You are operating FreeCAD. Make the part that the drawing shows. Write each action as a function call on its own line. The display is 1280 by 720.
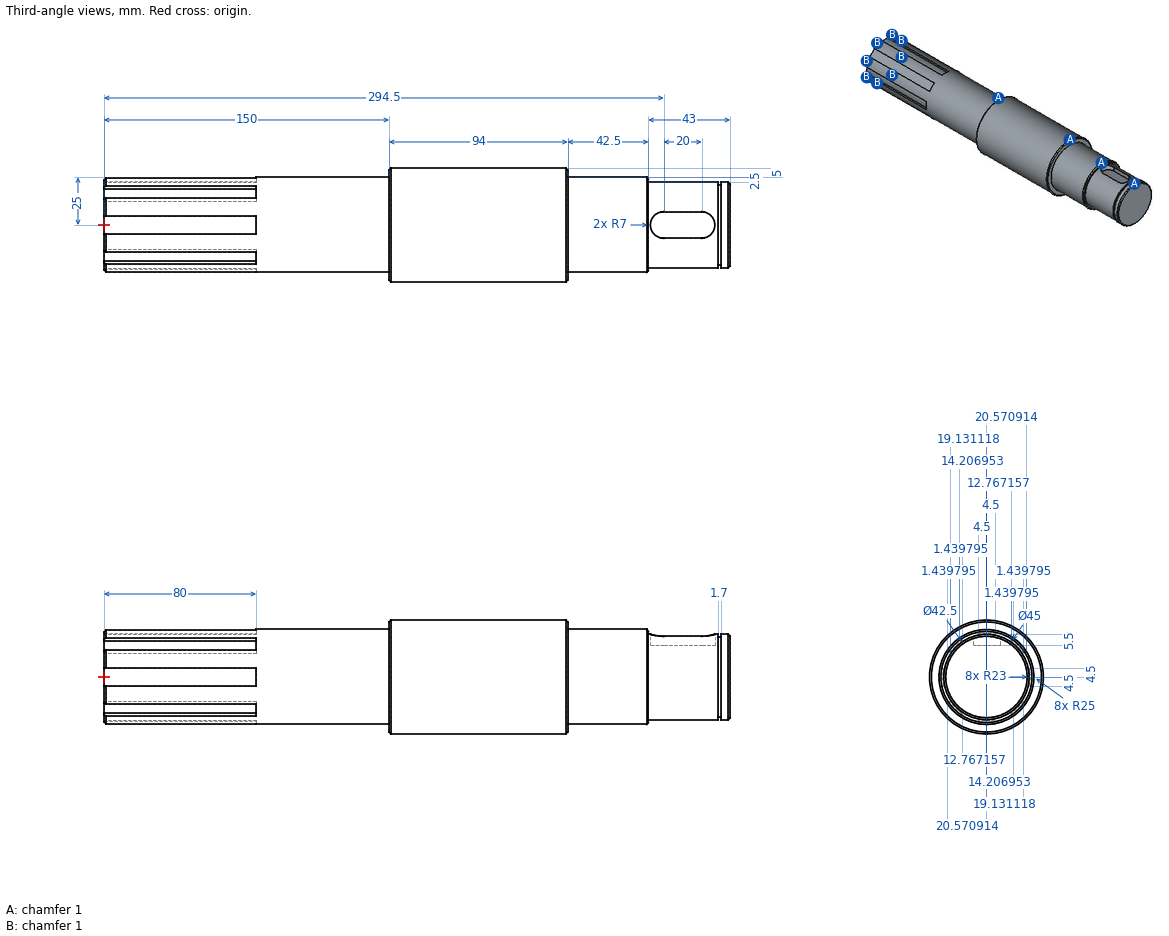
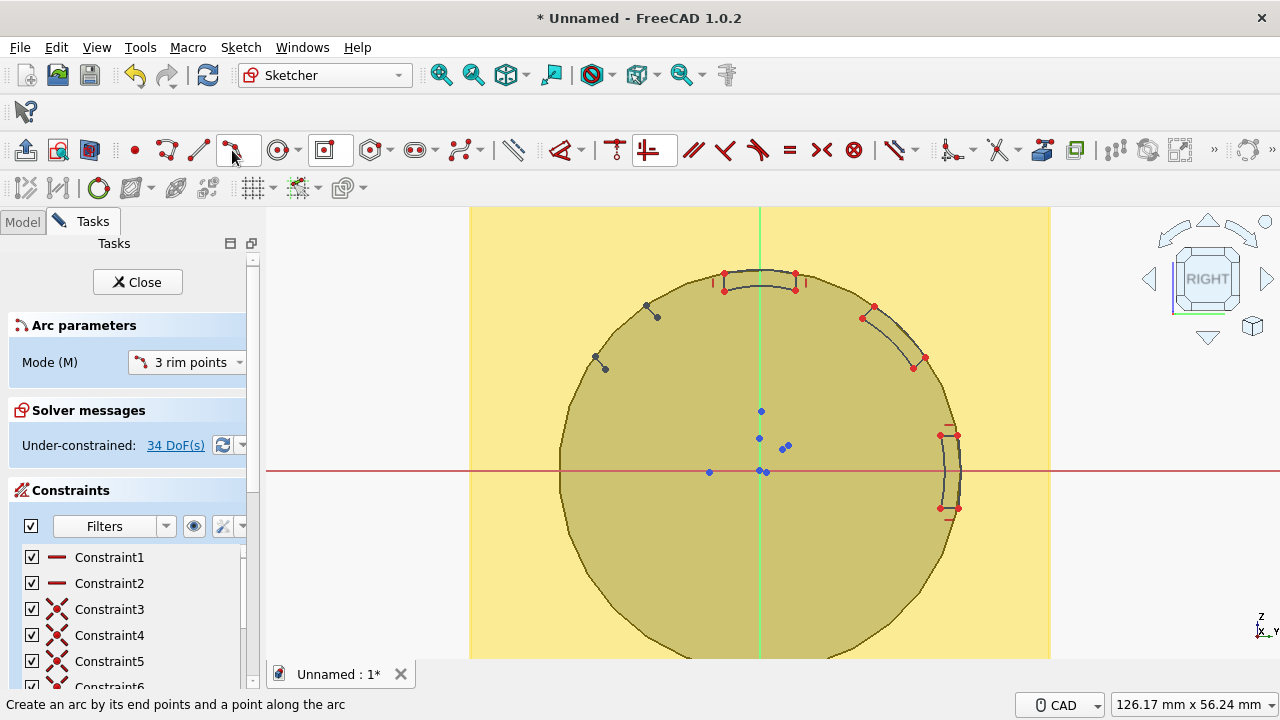
scroll(595, 356, up, 4)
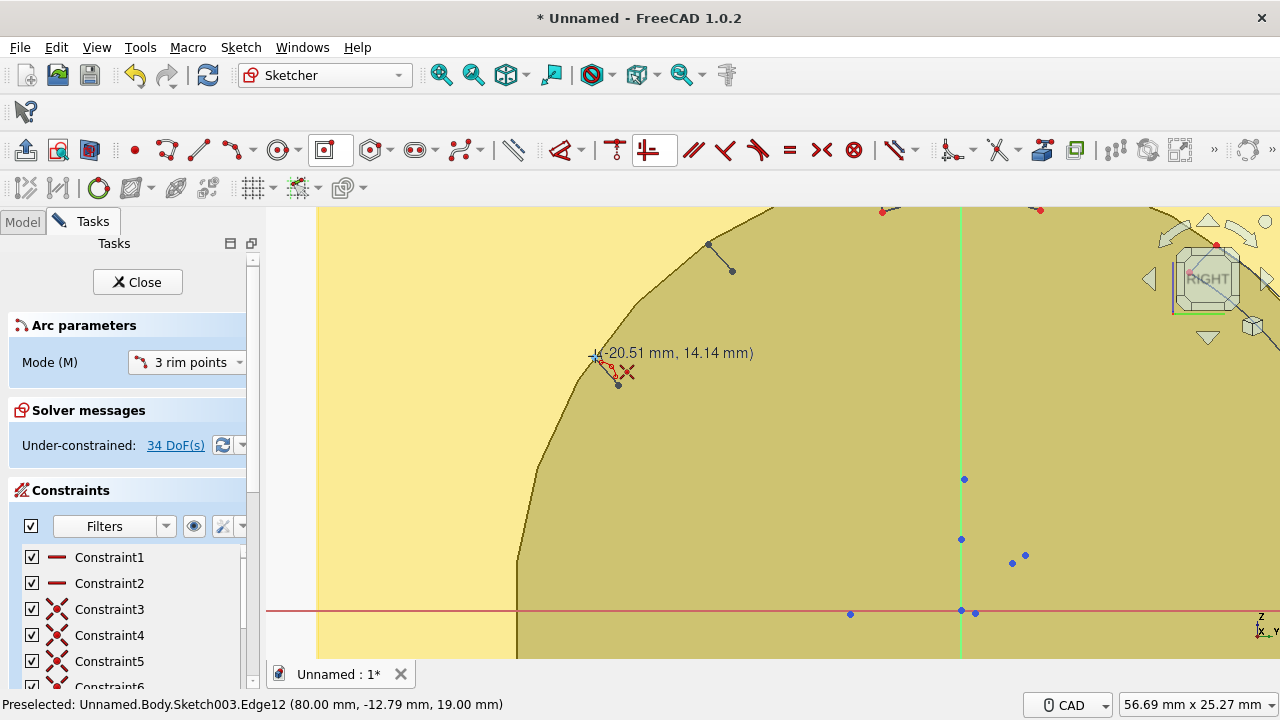
click(595, 358)
click(708, 244)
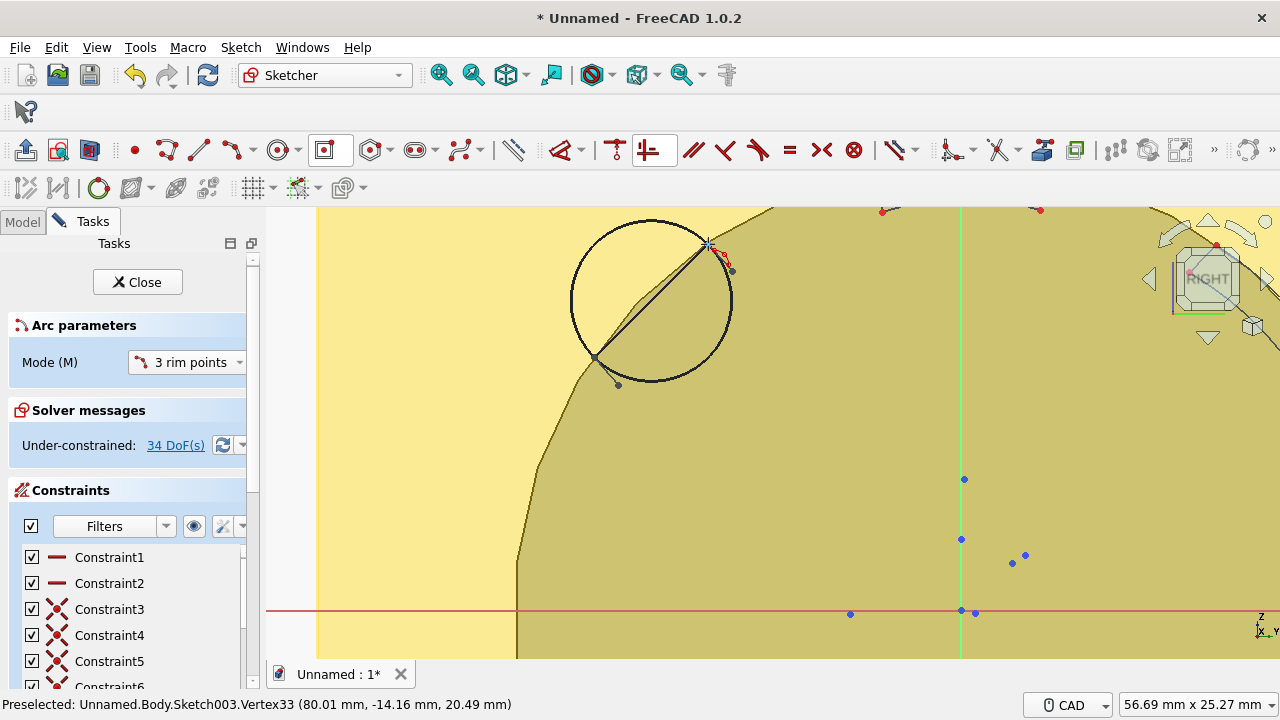
scroll(645, 295, up, 4)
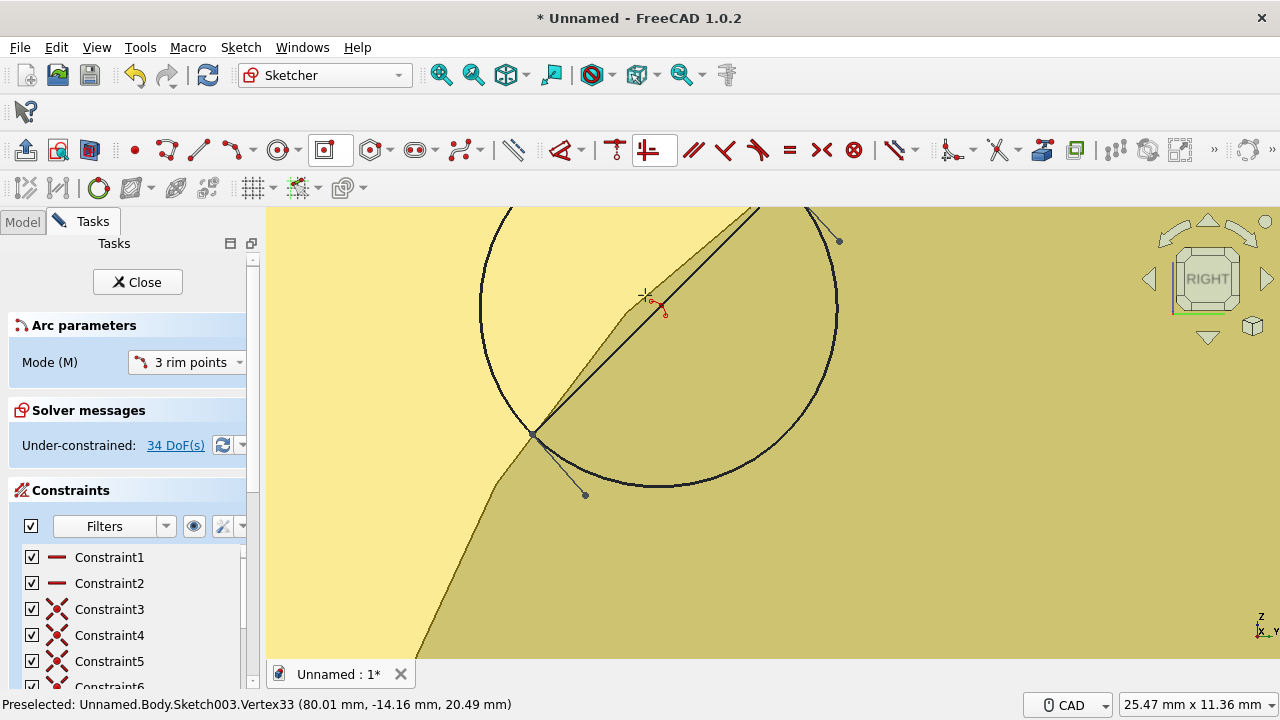
click(645, 294)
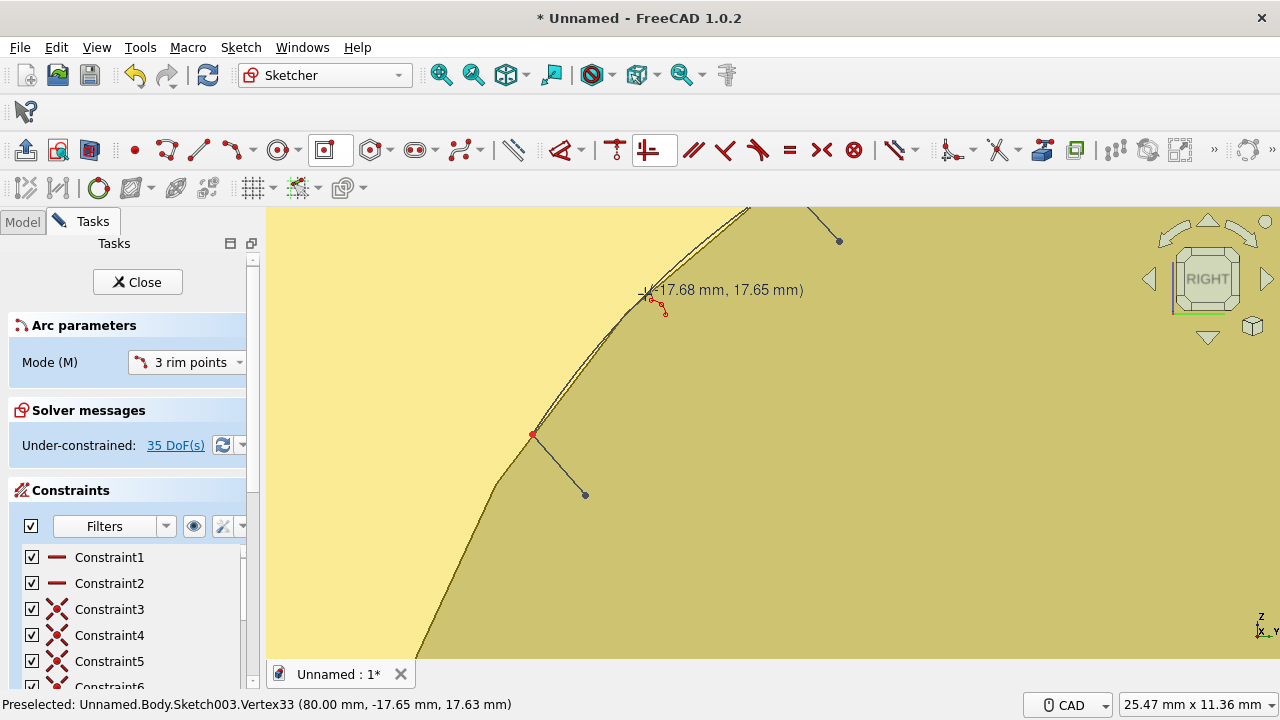
click(839, 241)
click(586, 495)
click(701, 350)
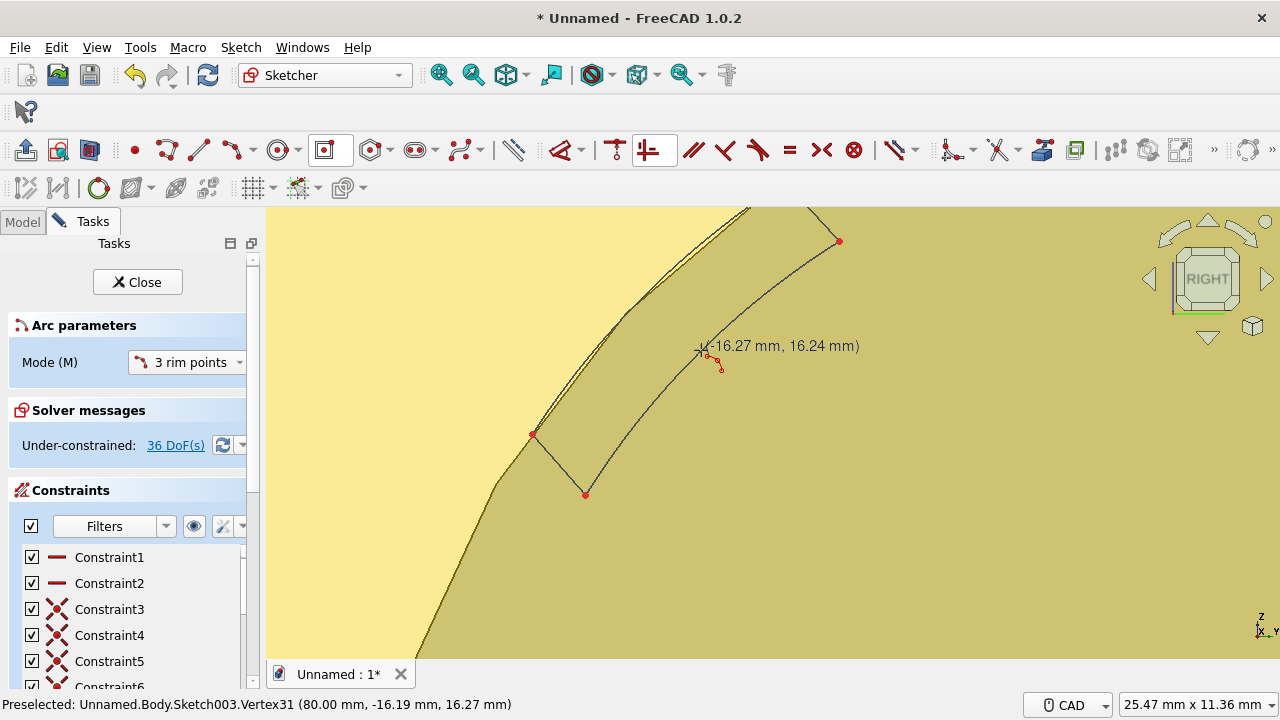
click(200, 150)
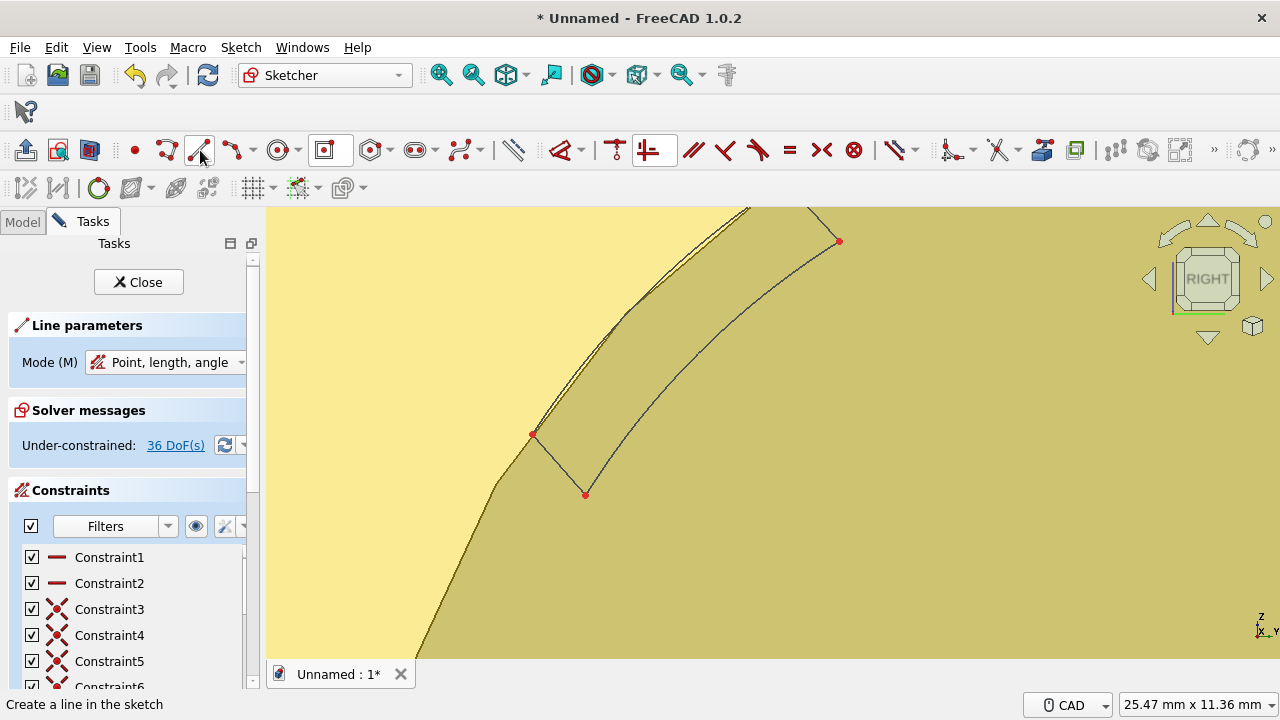
scroll(604, 345, down, 10)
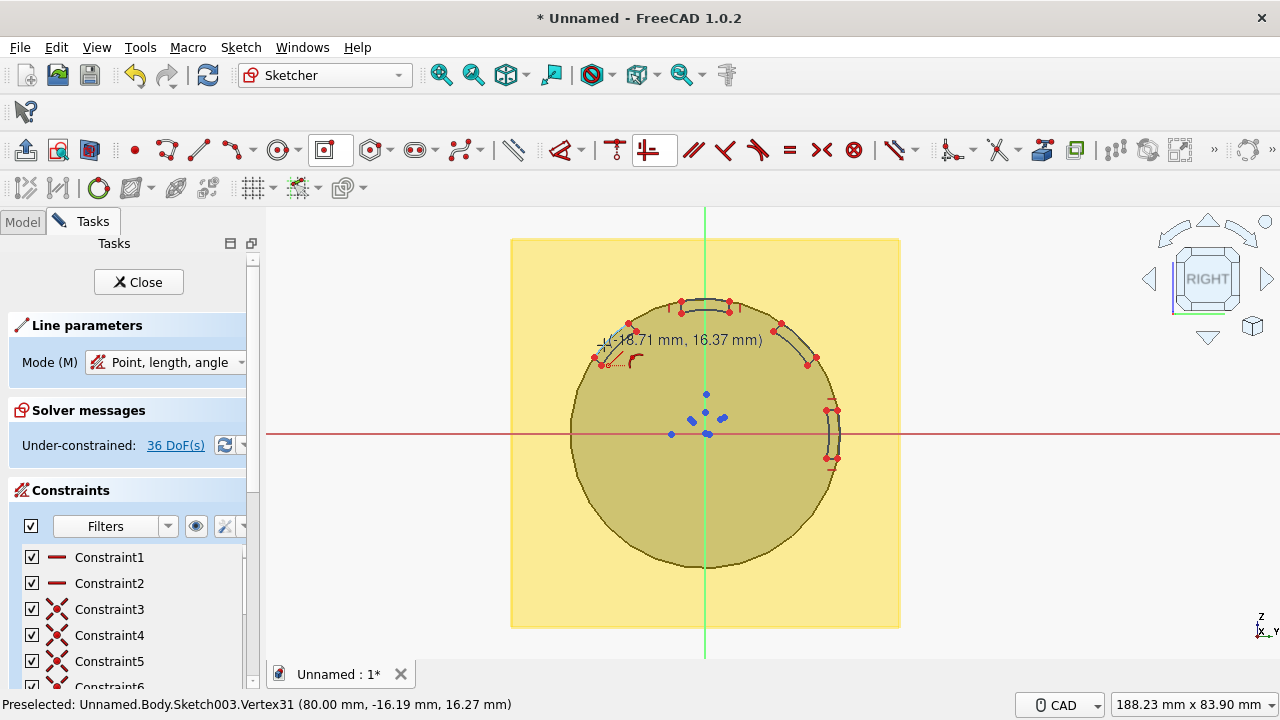
click(584, 458)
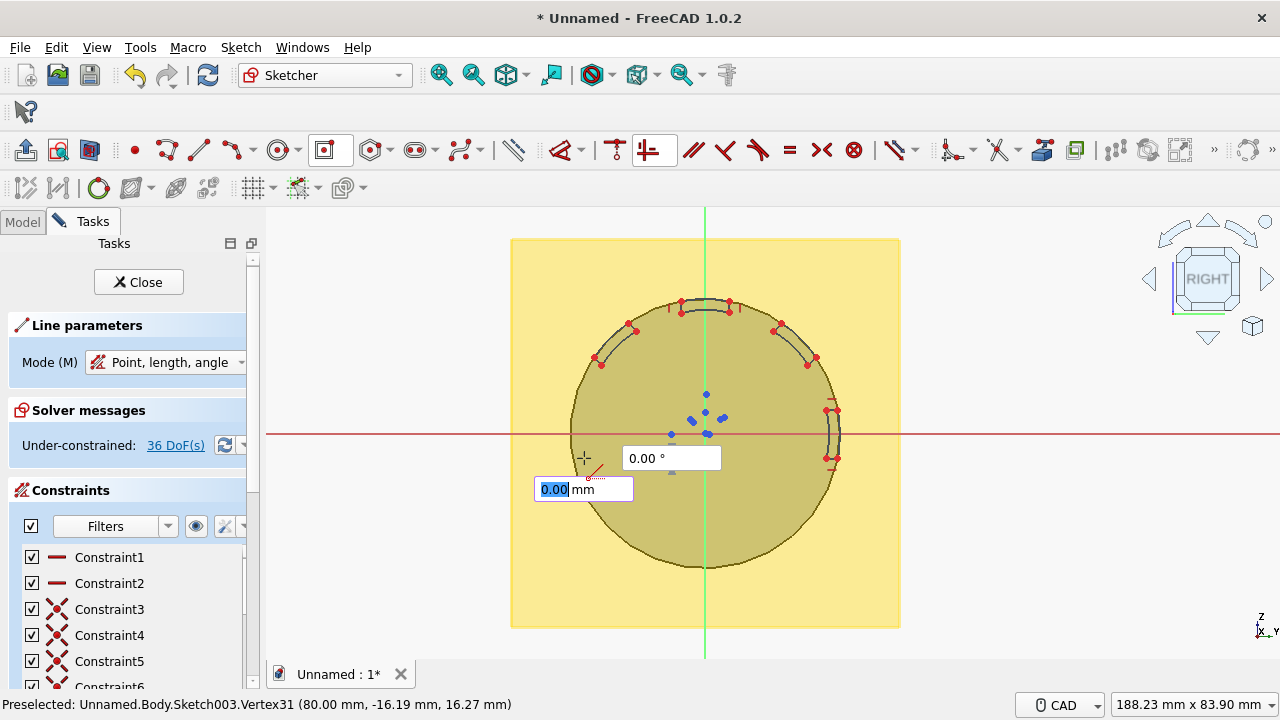
scroll(573, 458, up, 2)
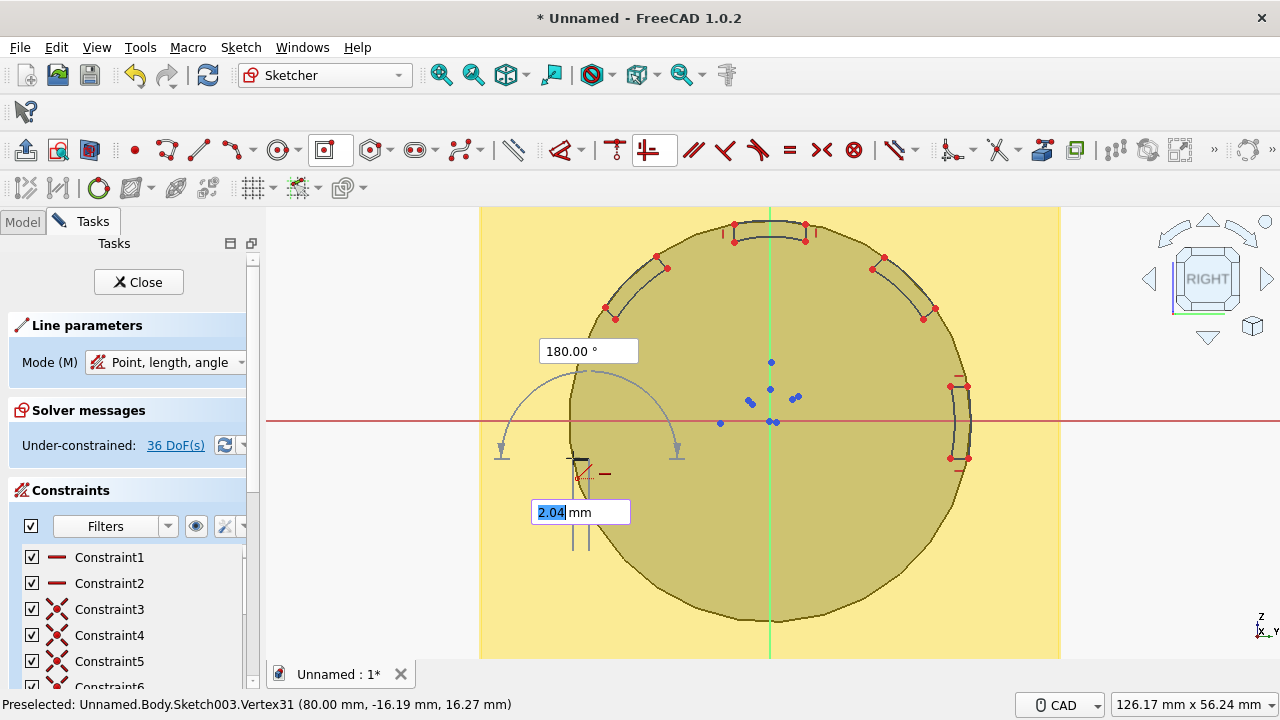
click(572, 458)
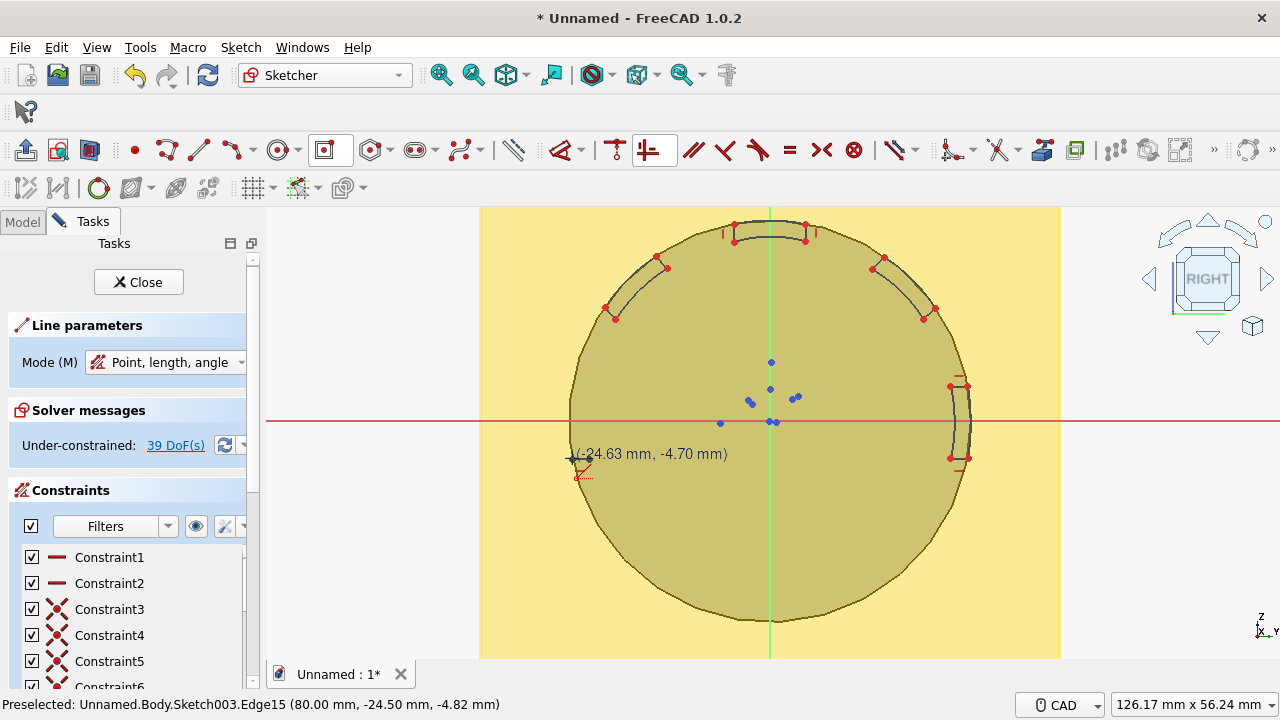
click(572, 385)
click(589, 385)